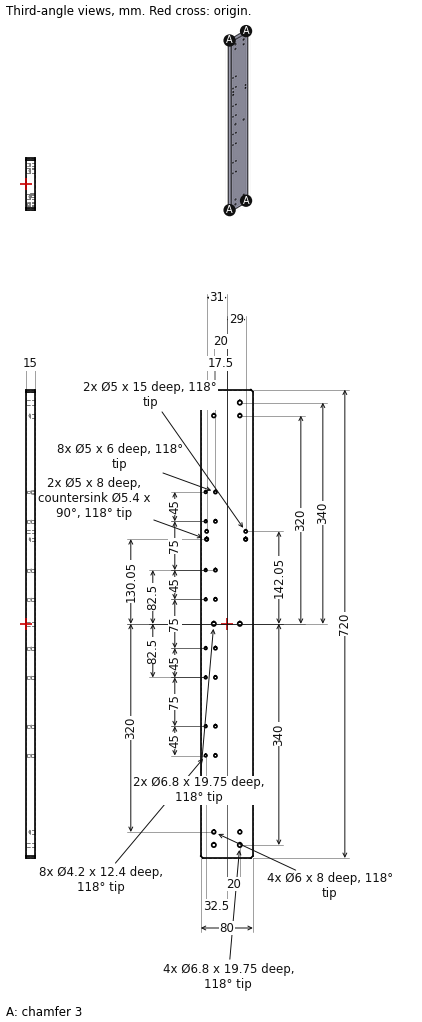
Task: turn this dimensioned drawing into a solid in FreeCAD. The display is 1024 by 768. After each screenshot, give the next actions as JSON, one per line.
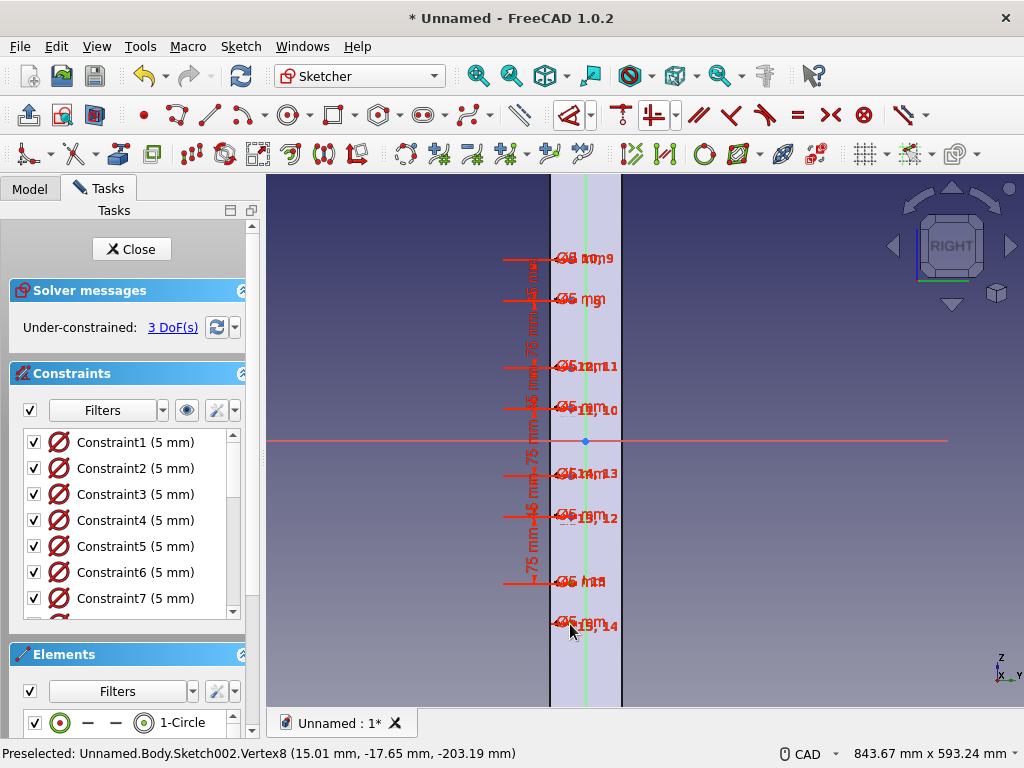
{"action": "left_click", "coordinate": [590, 116]}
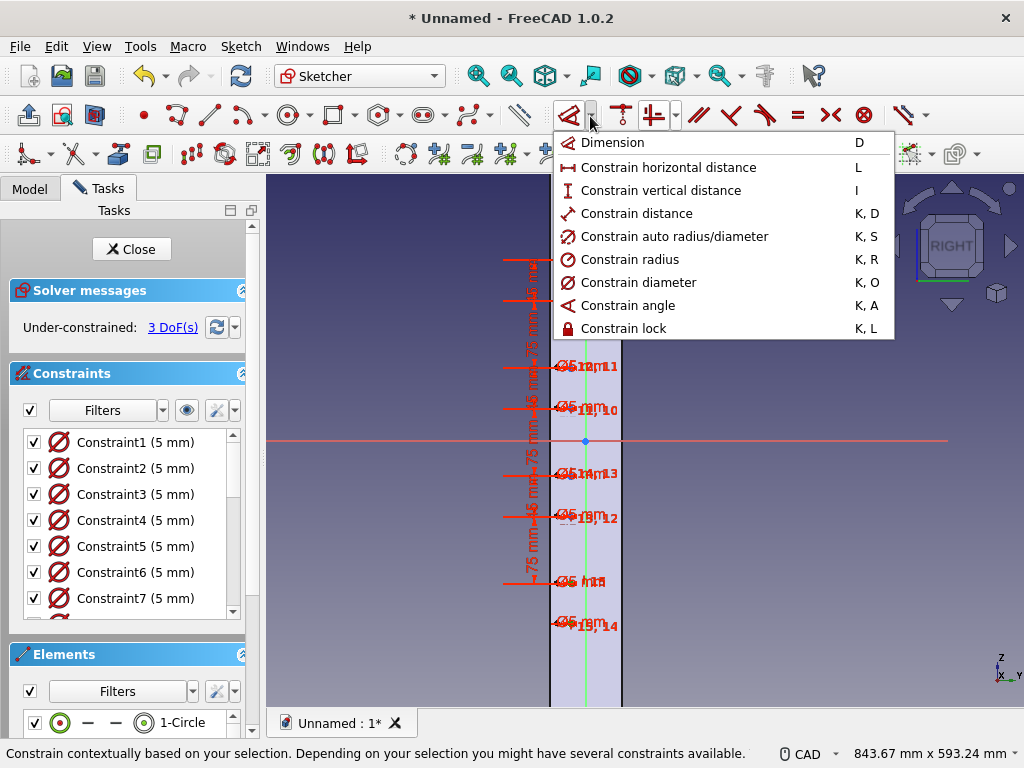
{"action": "left_click", "coordinate": [724, 190]}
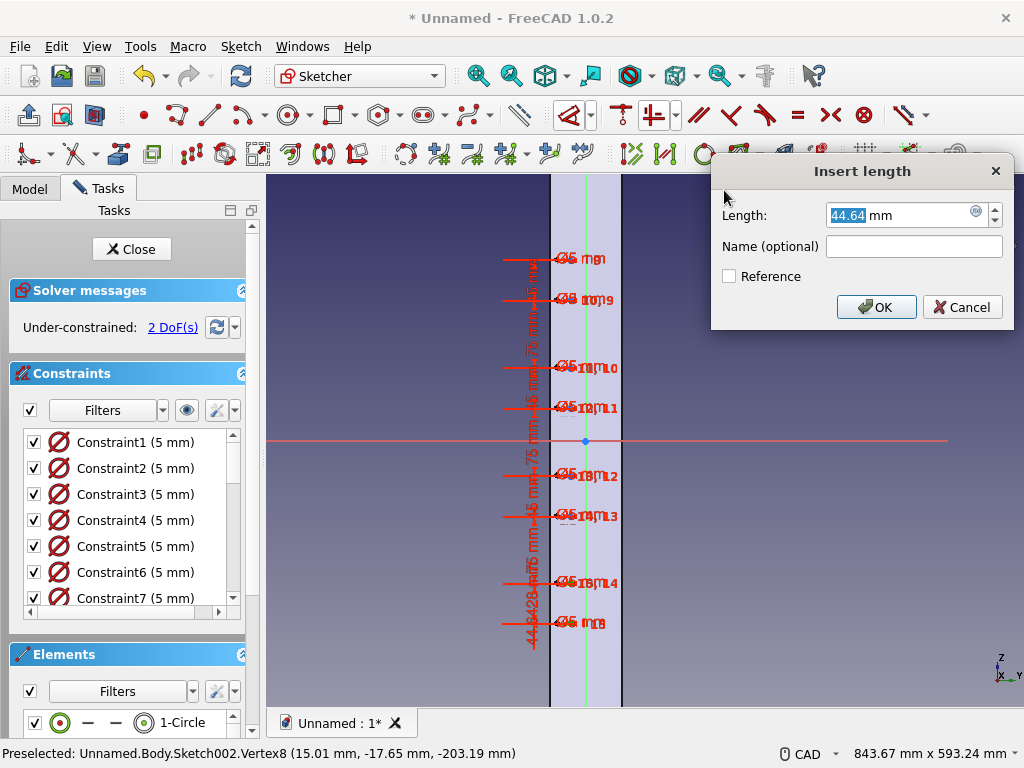
{"action": "type", "text": "45"}
{"action": "key", "text": "Return"}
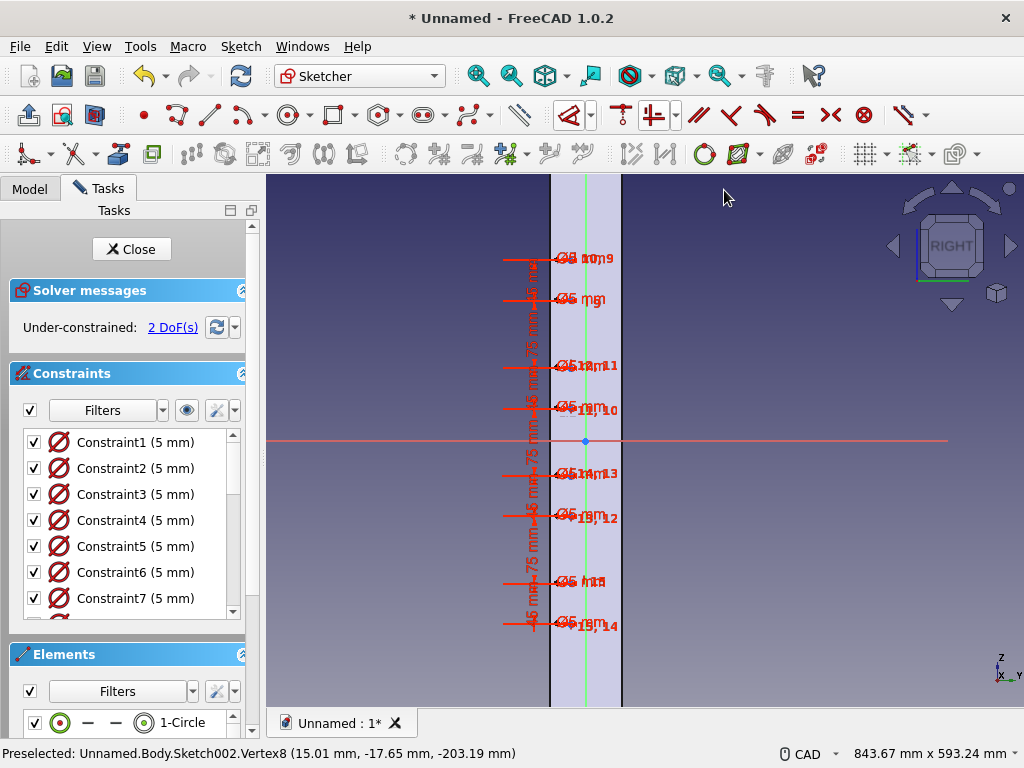
{"action": "scroll", "coordinate": [570, 260], "scroll_direction": "up", "scroll_amount": 5}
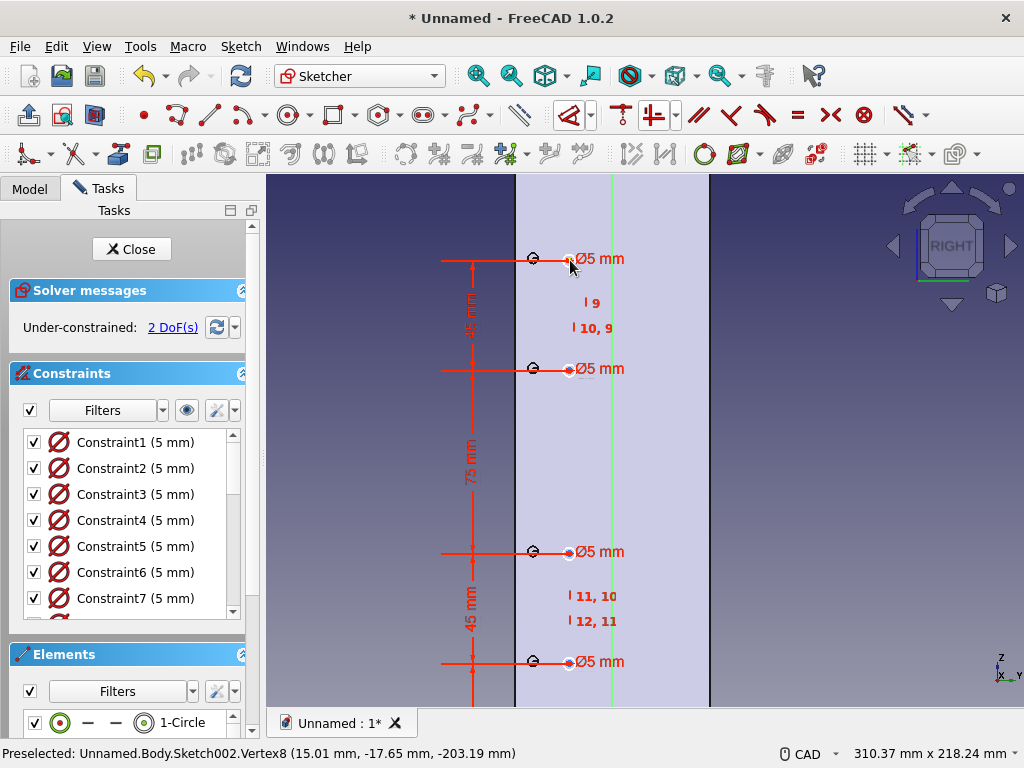
{"action": "left_click", "coordinate": [569, 261]}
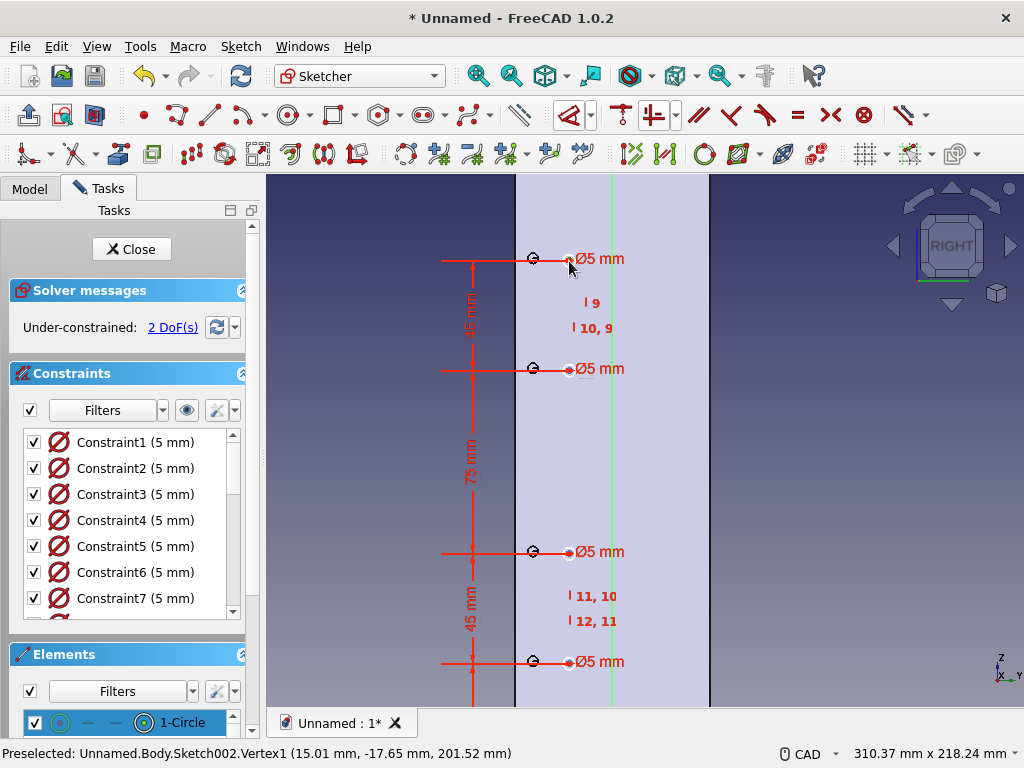
{"action": "key", "text": "l"}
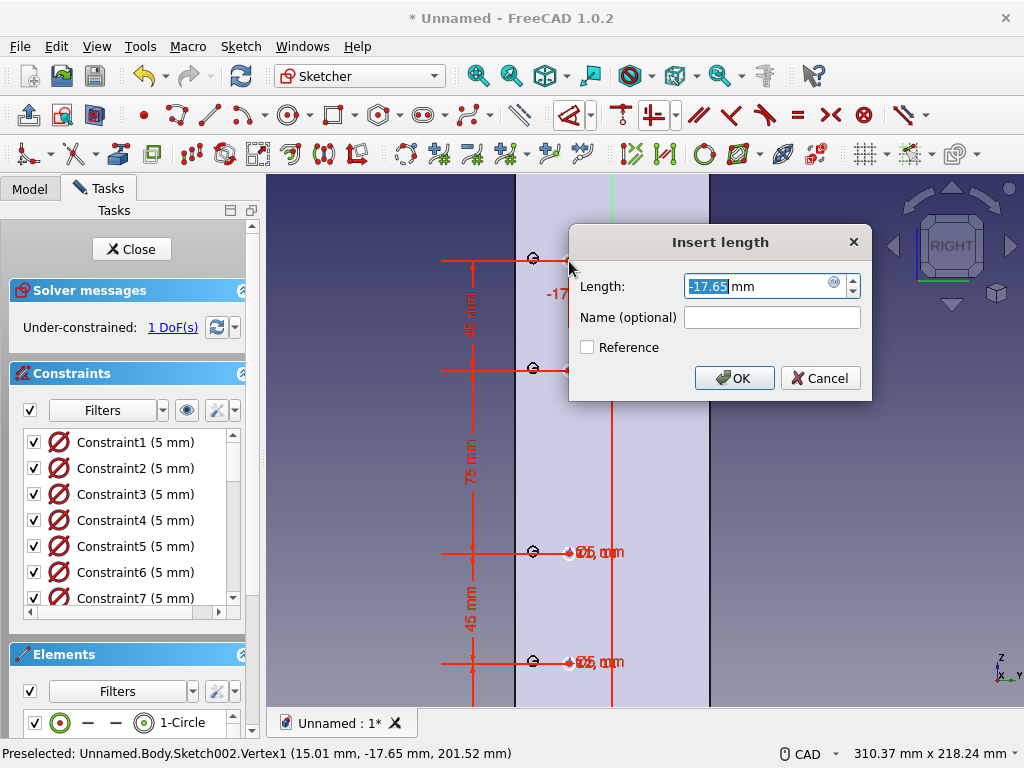
{"action": "type", "text": "-17.5"}
{"action": "key", "text": "Return"}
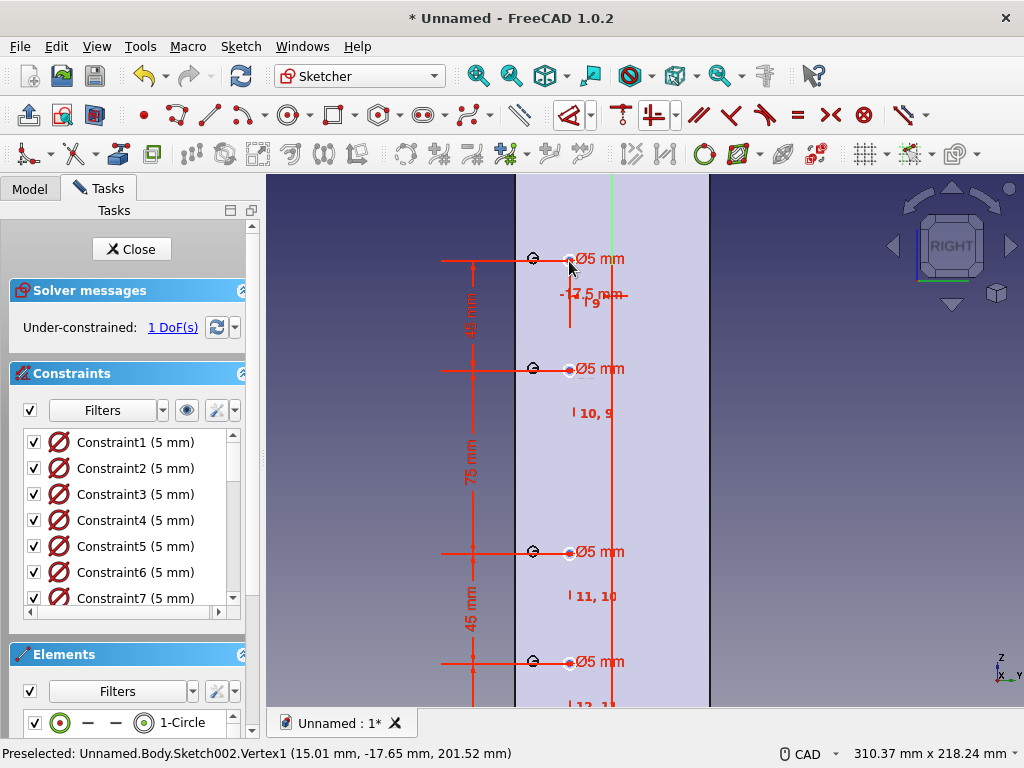
{"action": "left_click", "coordinate": [570, 554]}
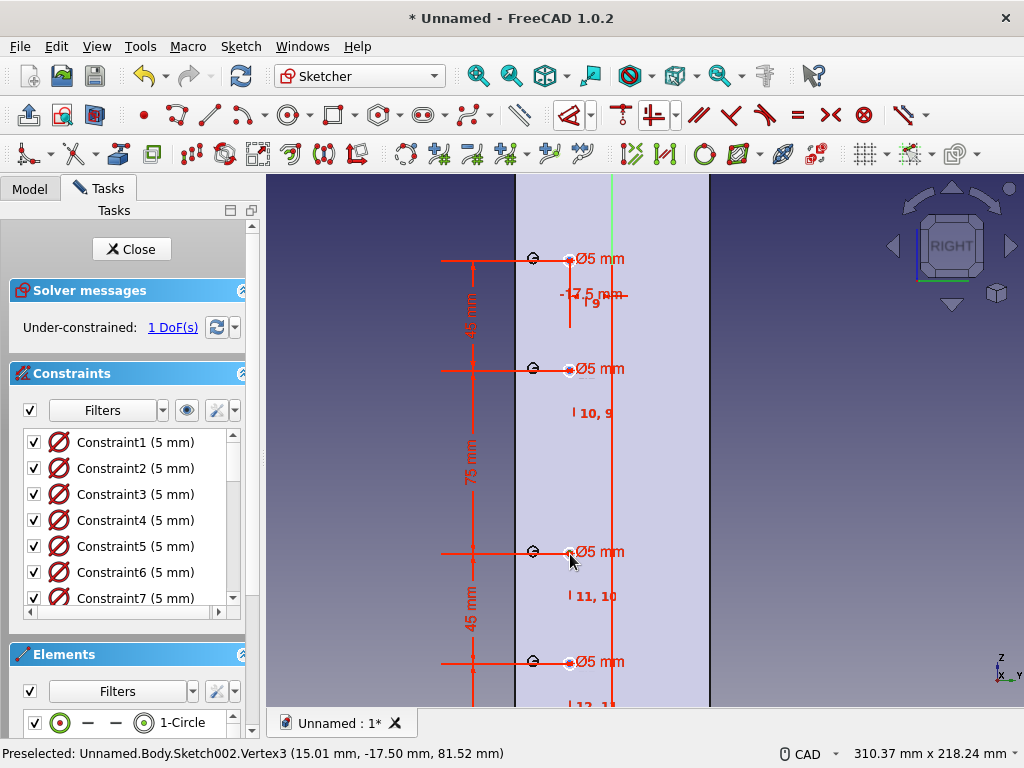
{"action": "key", "text": "i"}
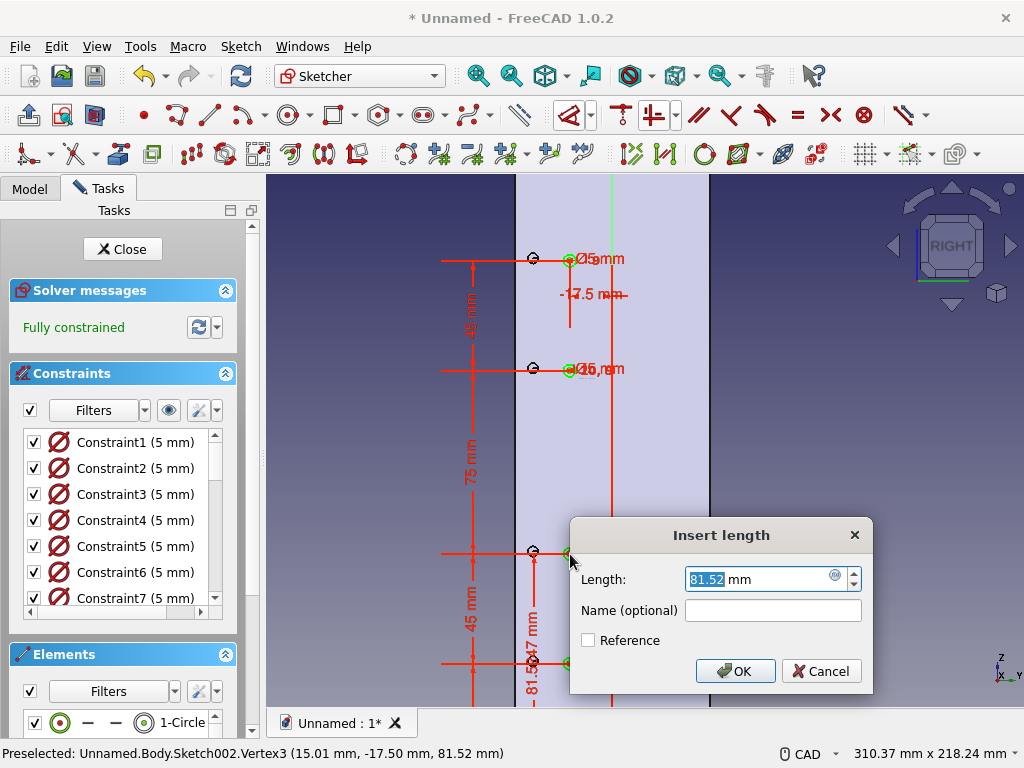
{"action": "type", "text": "82.5"}
{"action": "key", "text": "Return"}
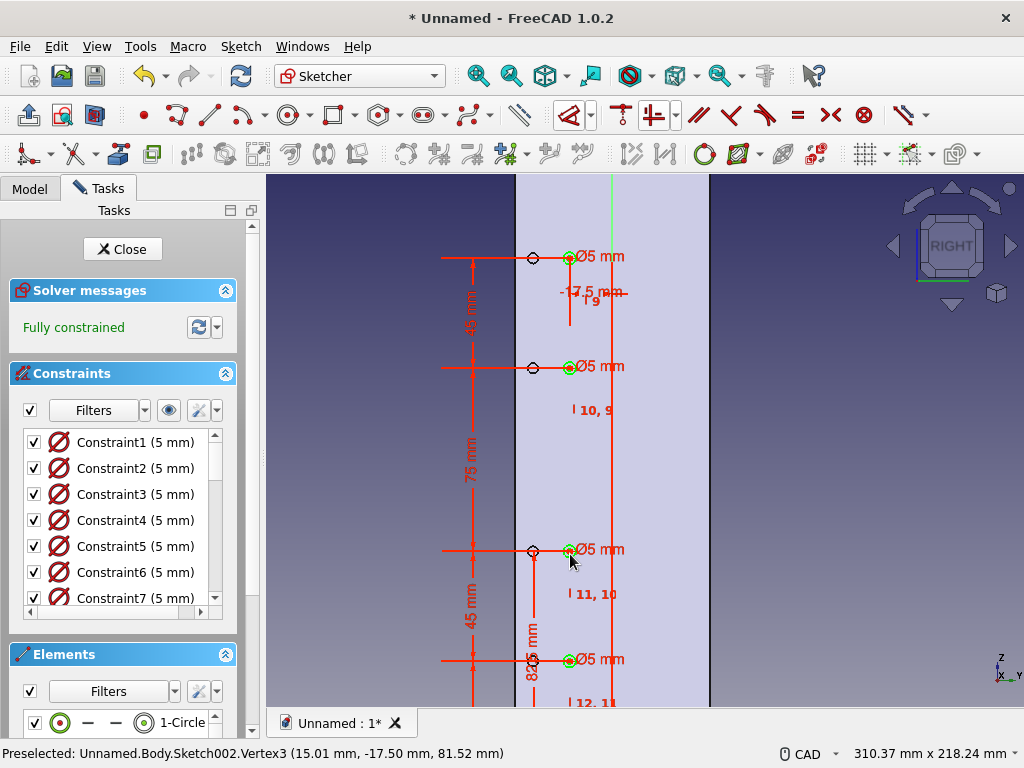
{"action": "left_click", "coordinate": [123, 249]}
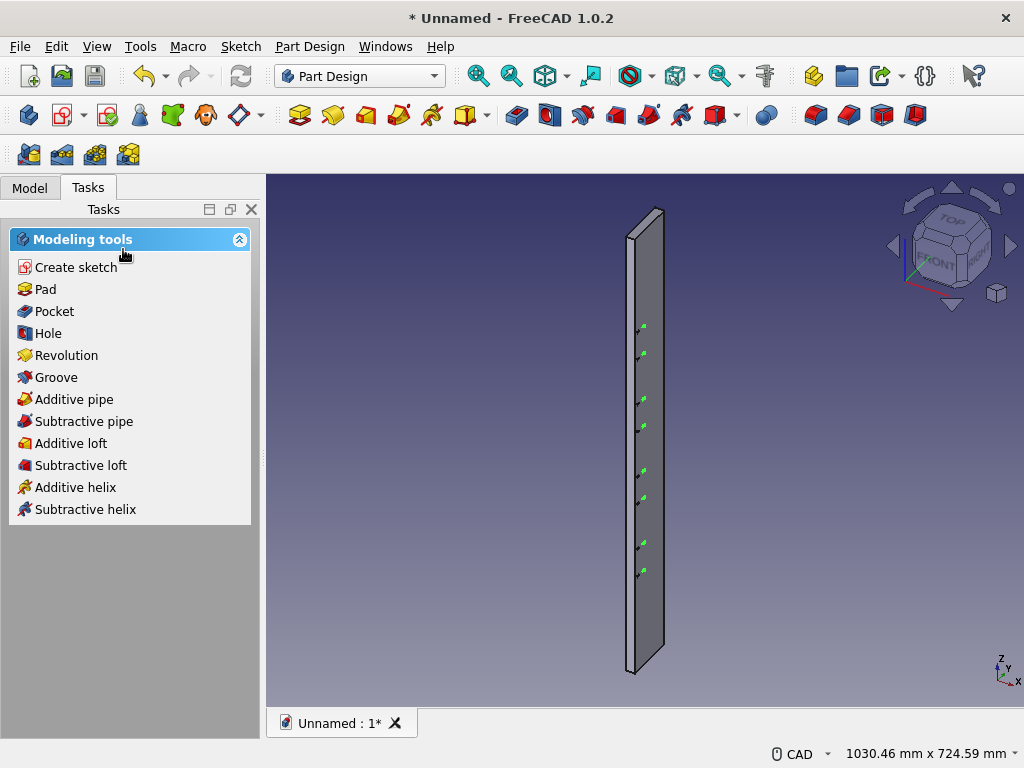
{"action": "left_click", "coordinate": [550, 116]}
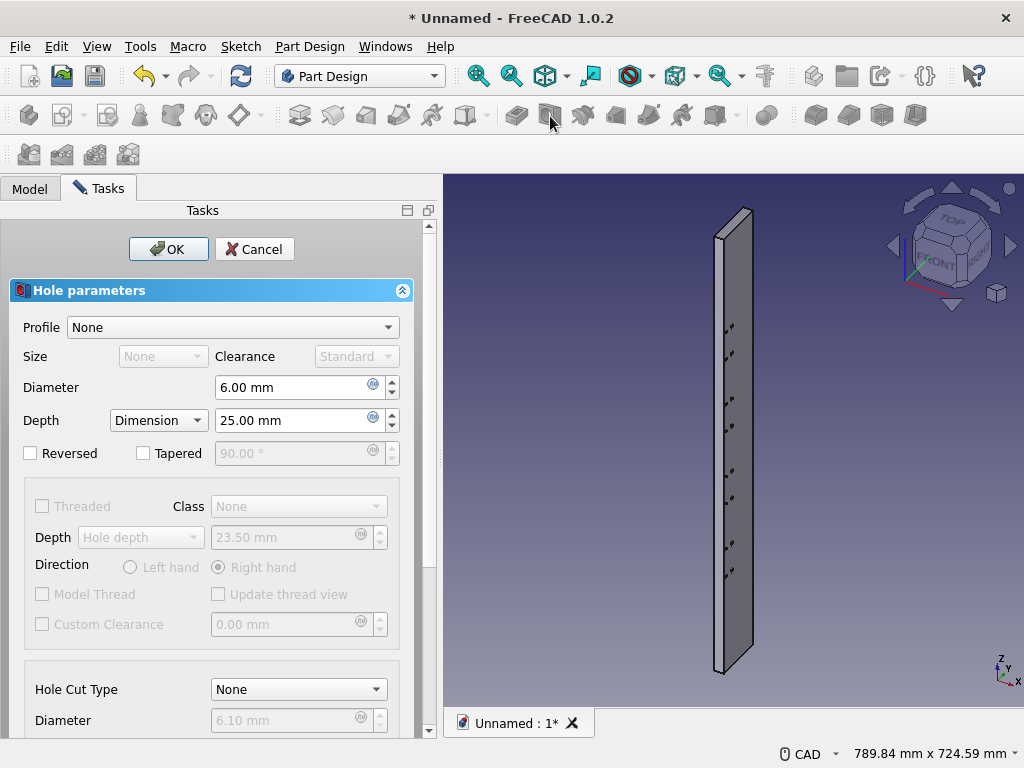
{"action": "triple_click", "coordinate": [300, 388]}